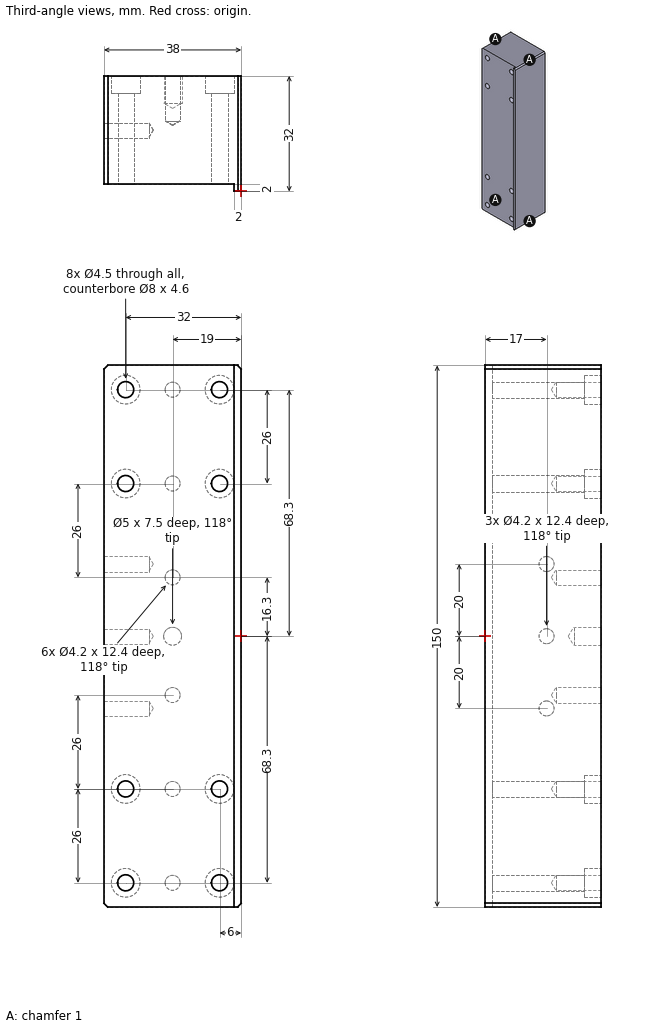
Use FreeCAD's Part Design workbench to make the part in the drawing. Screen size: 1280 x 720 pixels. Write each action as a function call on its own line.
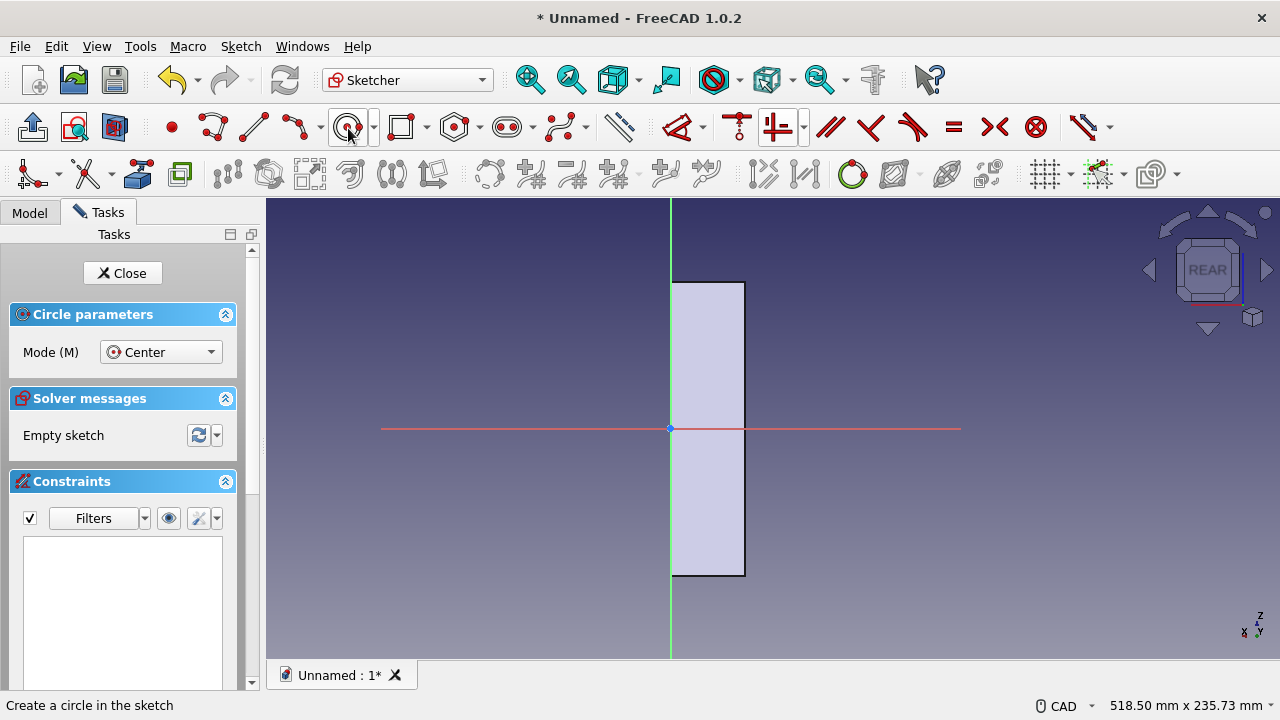
scroll(734, 295, up, 9)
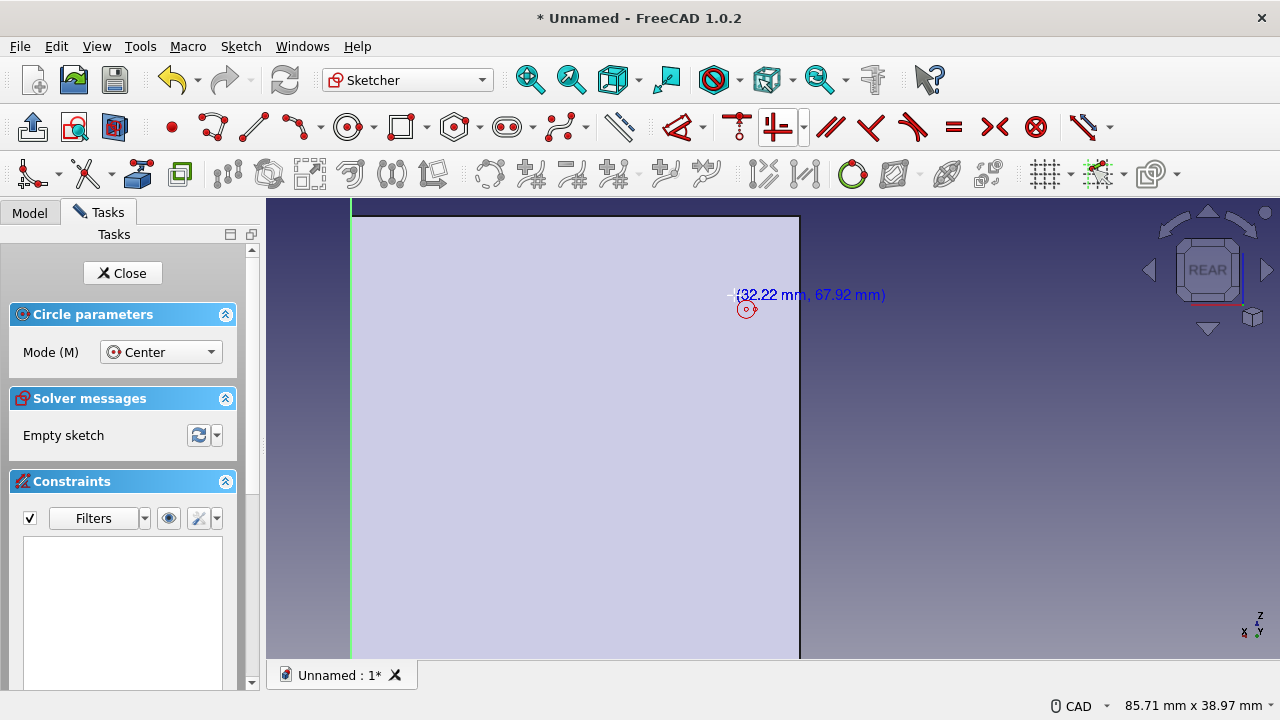
scroll(734, 295, down, 9)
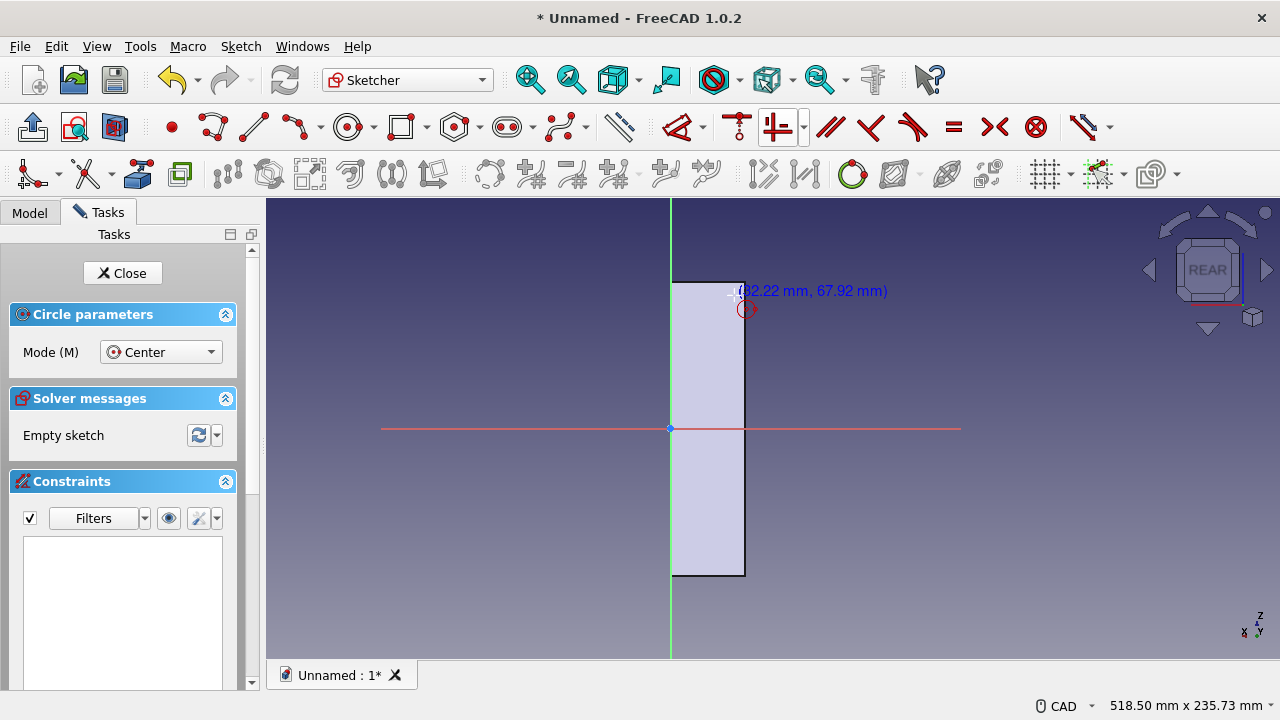
click(734, 295)
move(737, 292)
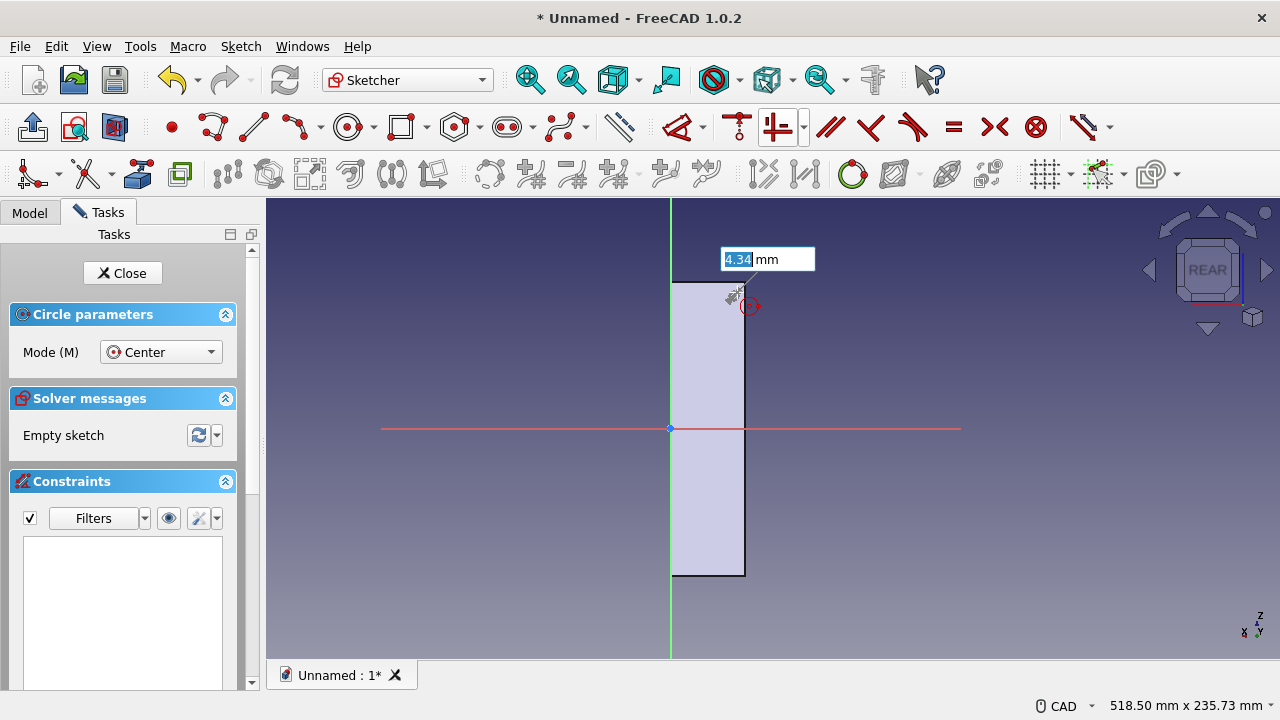
text(4.5)
key(Return)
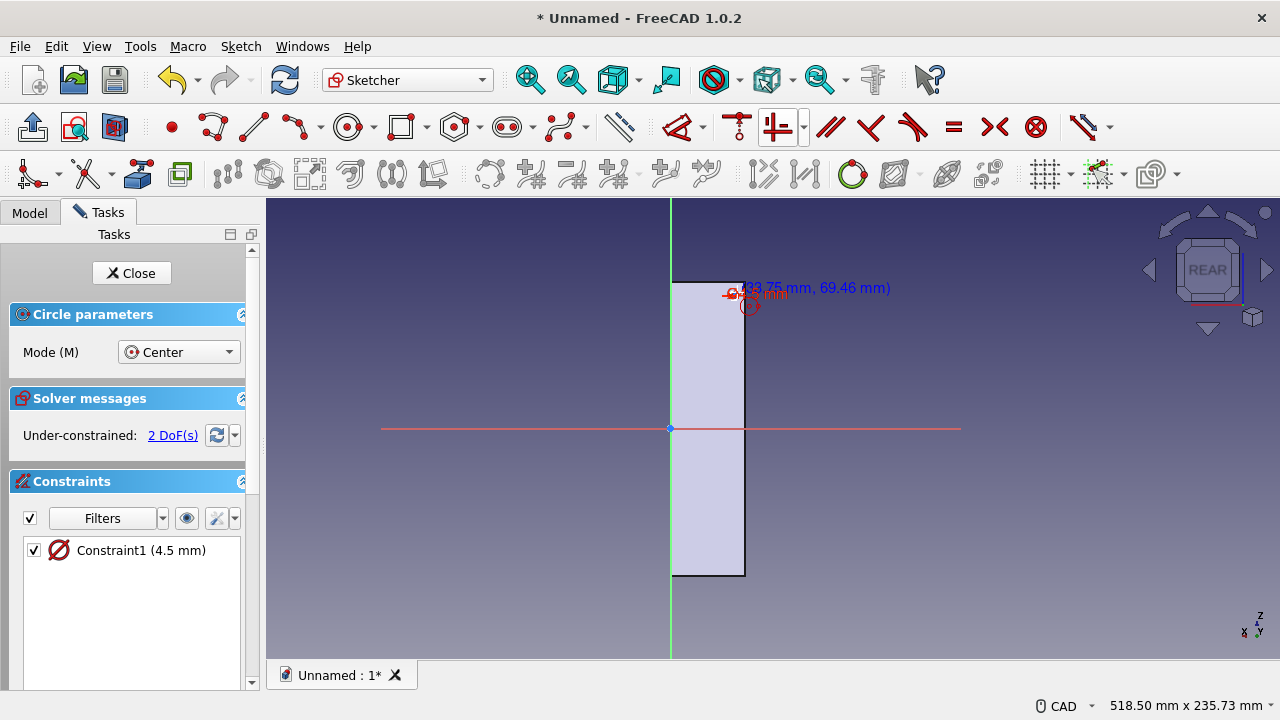
scroll(734, 562, up, 9)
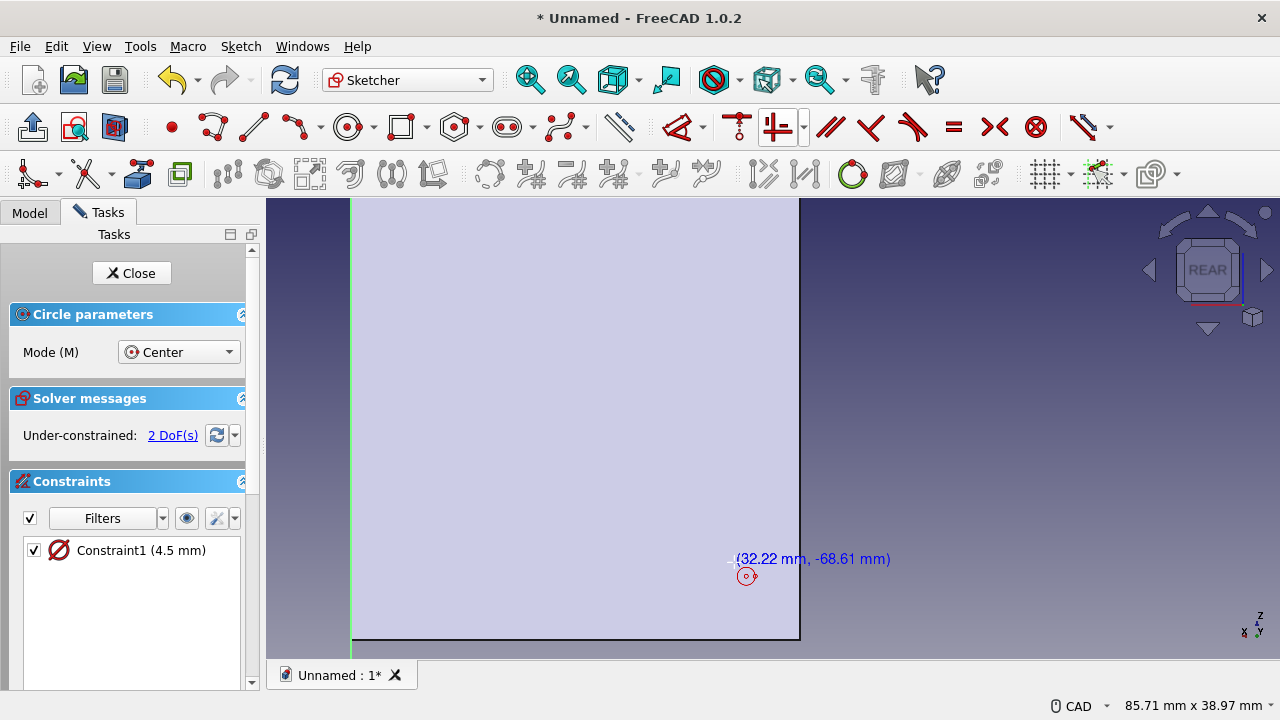
scroll(734, 562, down, 9)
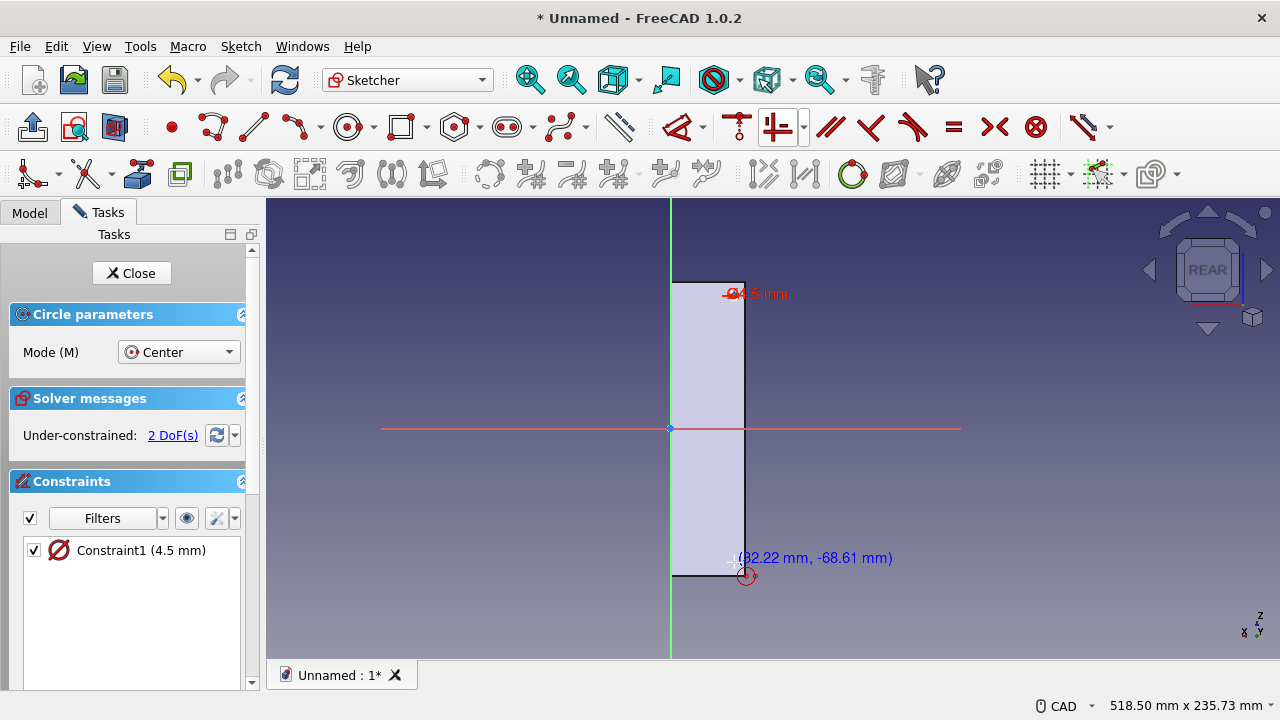
click(734, 562)
move(737, 559)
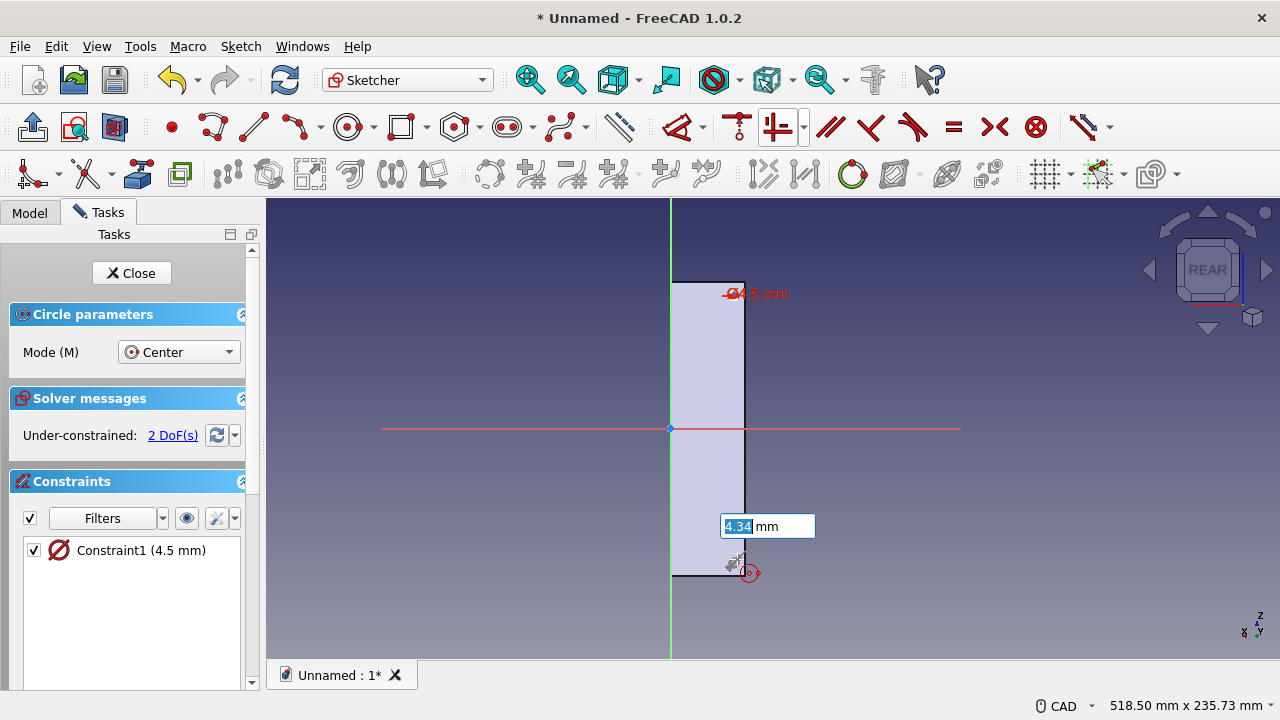
text(4.5)
key(Return)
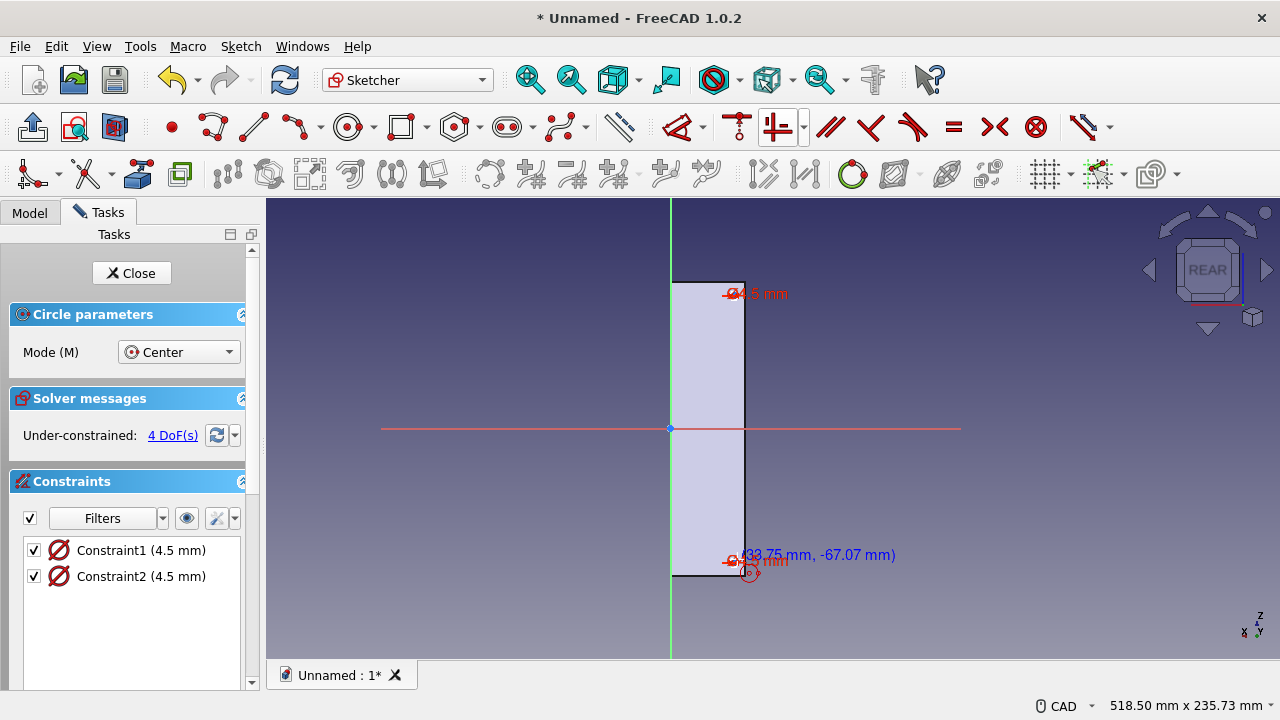
scroll(683, 512, up, 9)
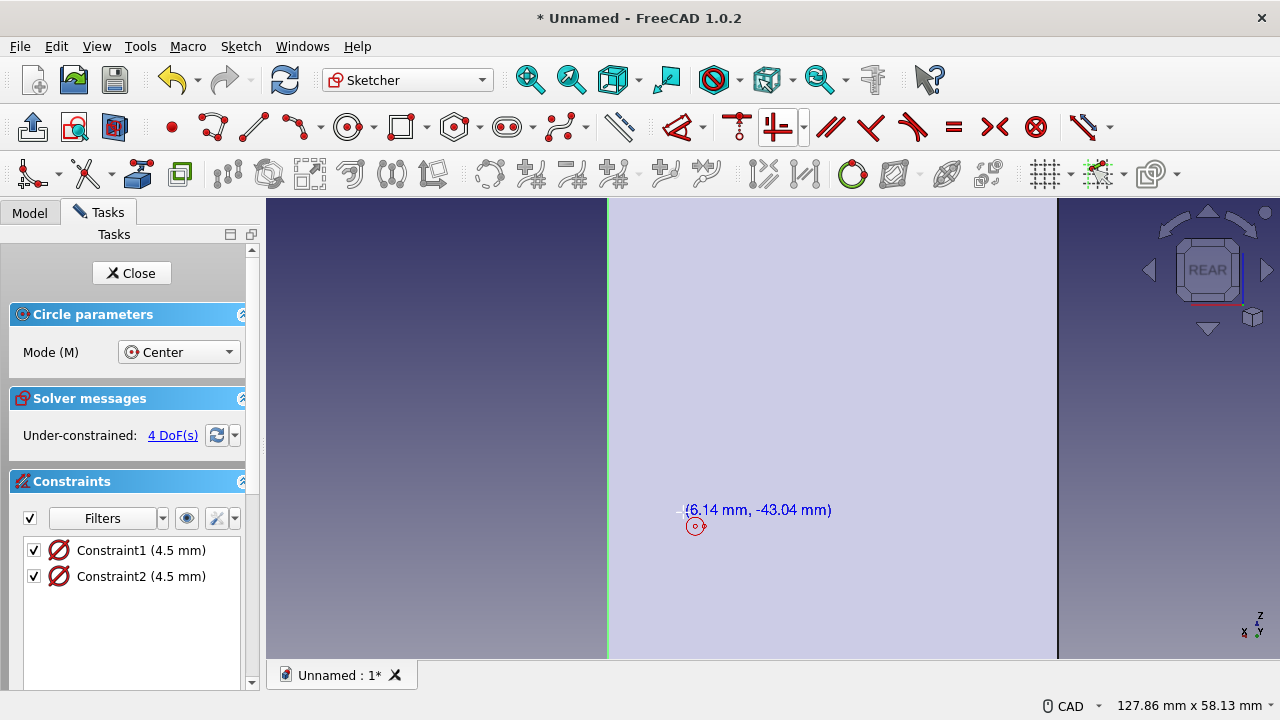
scroll(683, 512, down, 9)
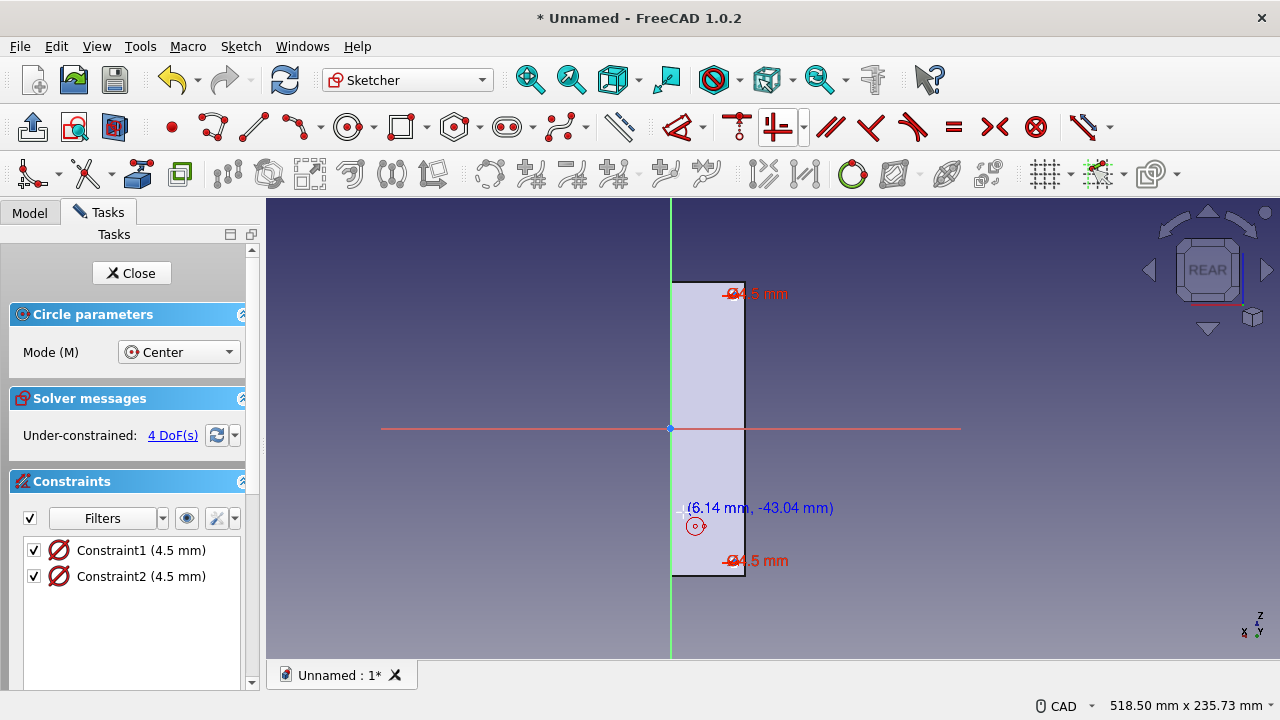
scroll(683, 512, up, 2)